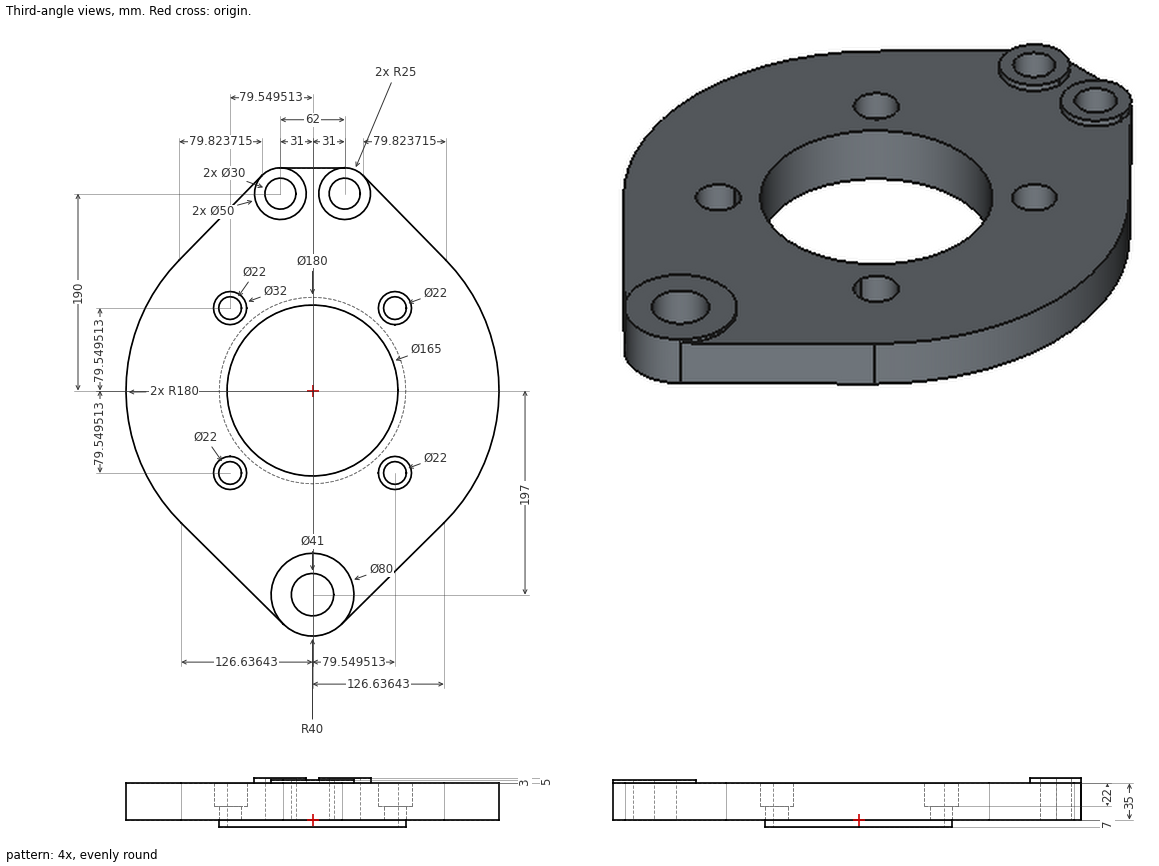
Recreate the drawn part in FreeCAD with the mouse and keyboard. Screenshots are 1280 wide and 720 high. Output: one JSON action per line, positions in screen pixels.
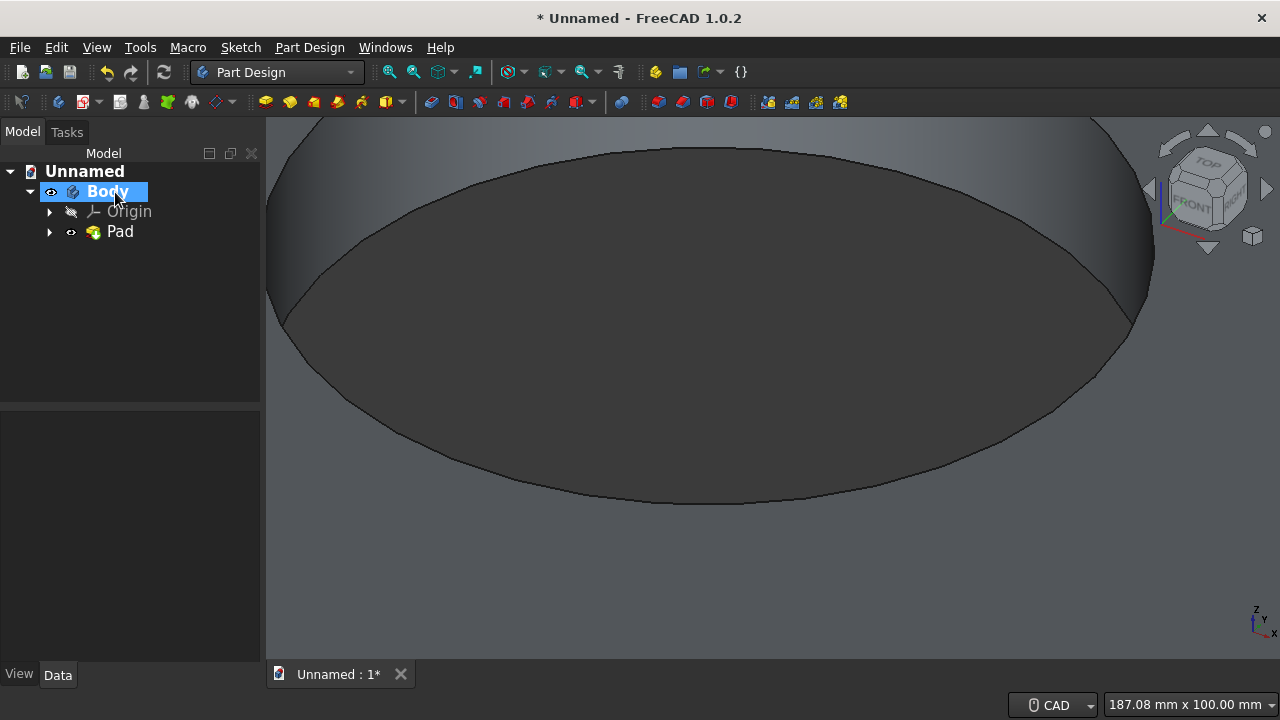
{"action": "key", "text": "v f"}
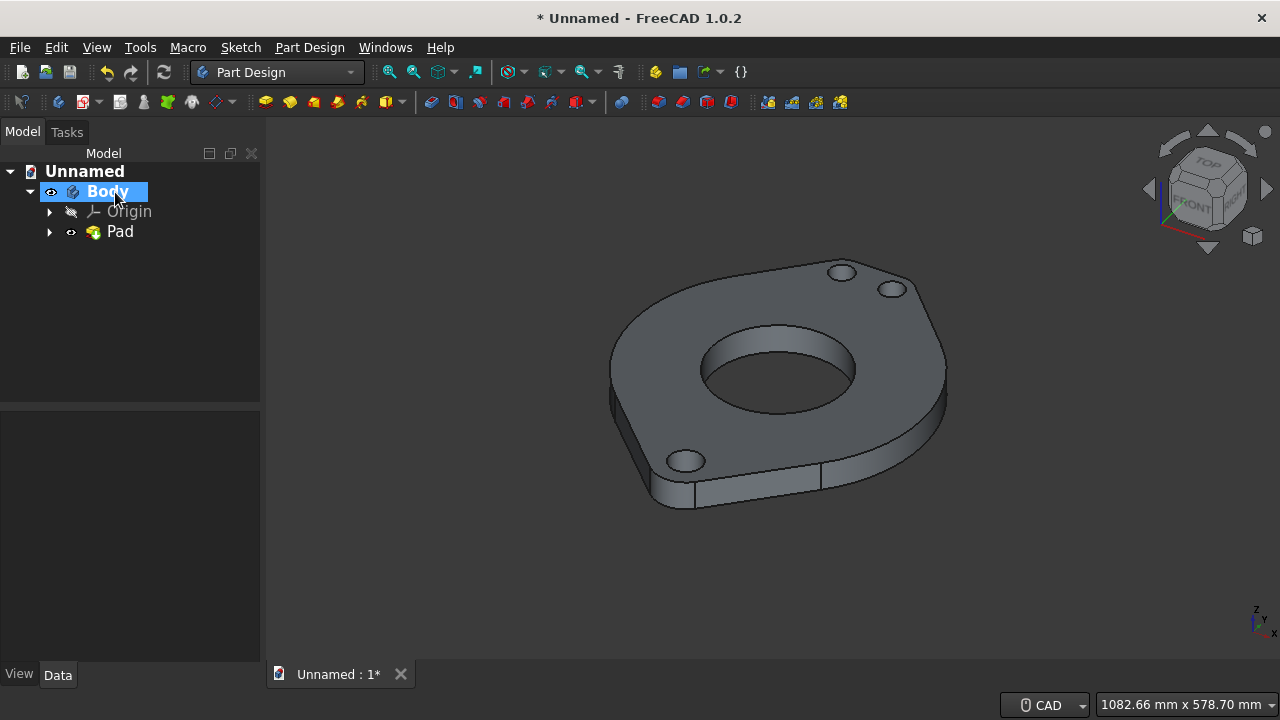
{"action": "left_click", "coordinate": [875, 327]}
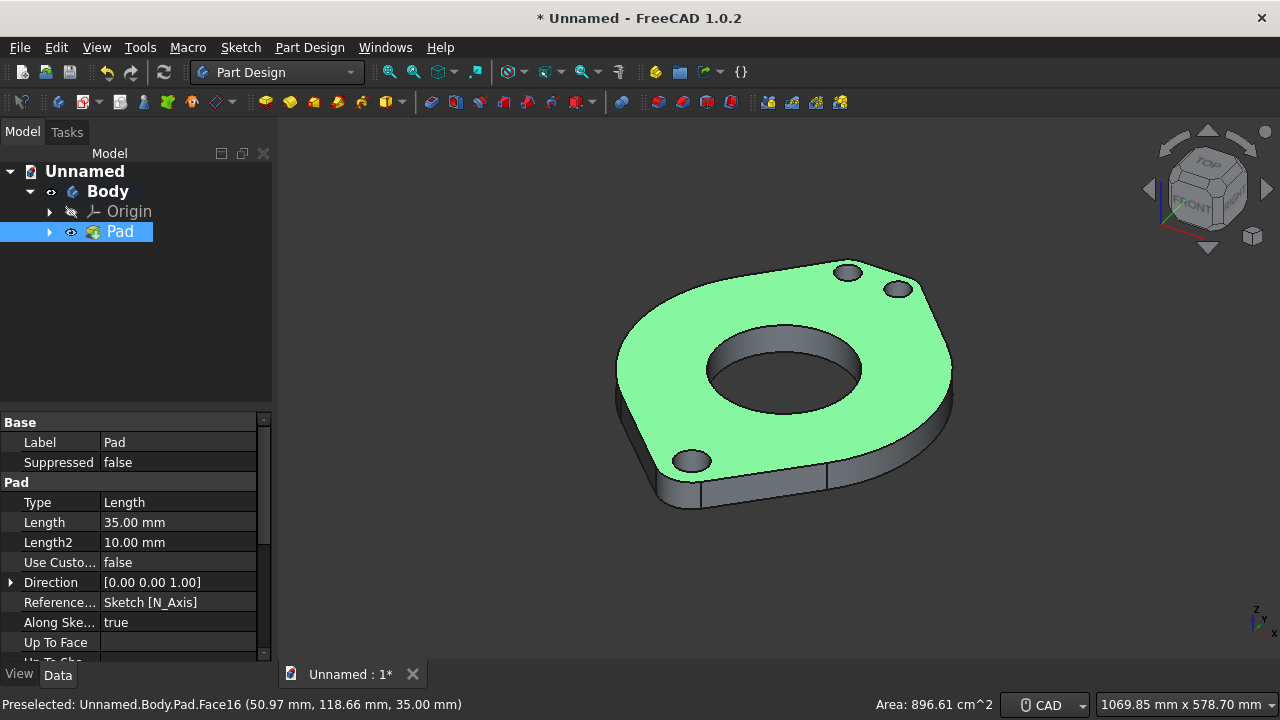
{"action": "left_click", "coordinate": [84, 102]}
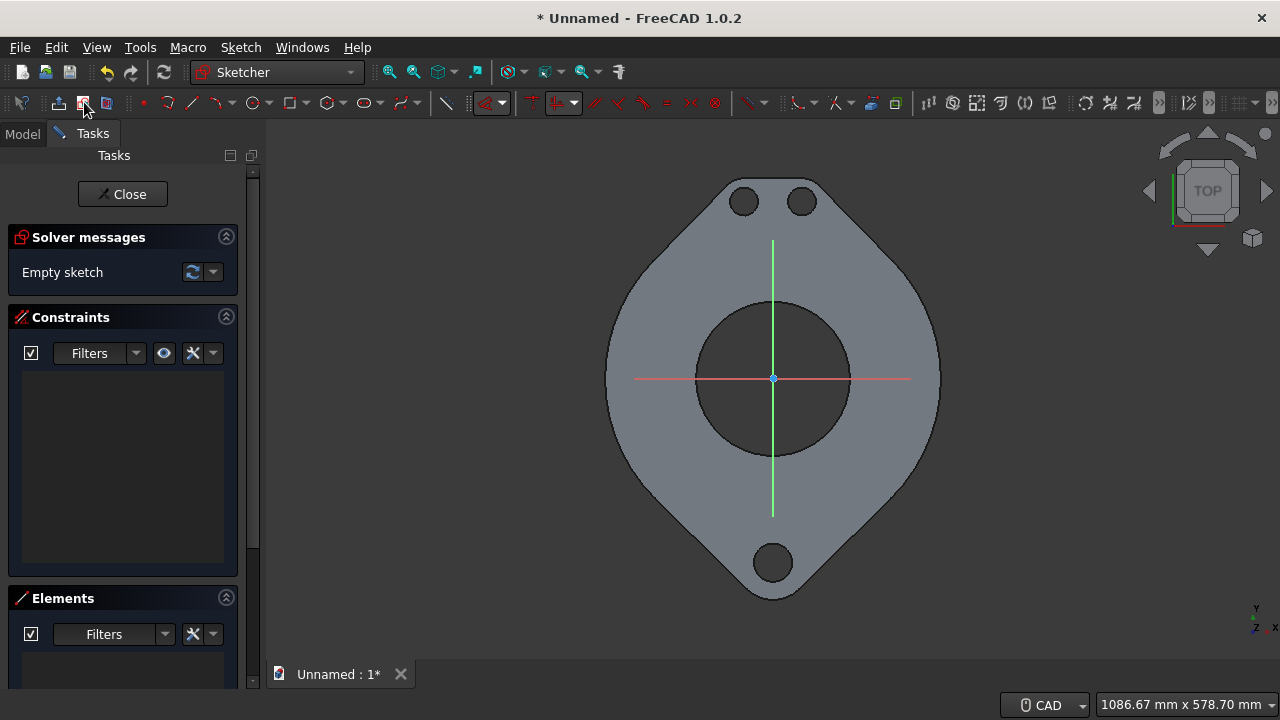
{"action": "scroll", "coordinate": [856, 147], "scroll_direction": "up", "scroll_amount": 3}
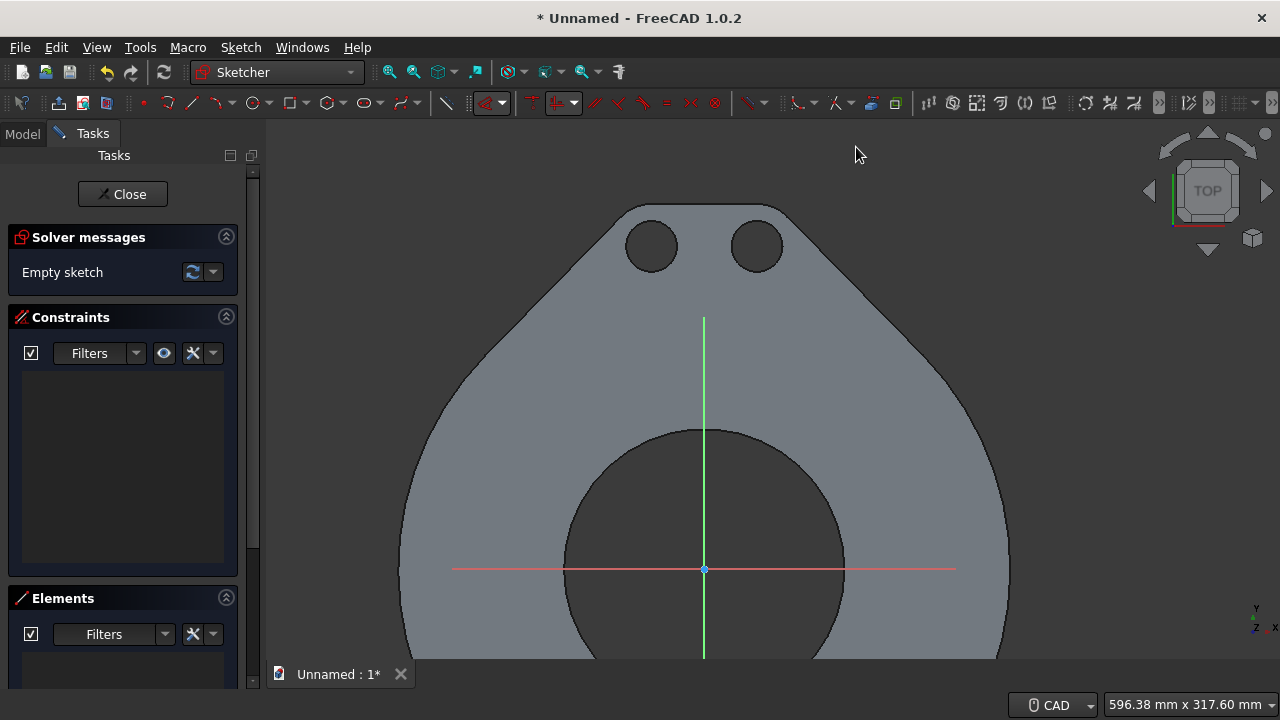
{"action": "left_click", "coordinate": [254, 104]}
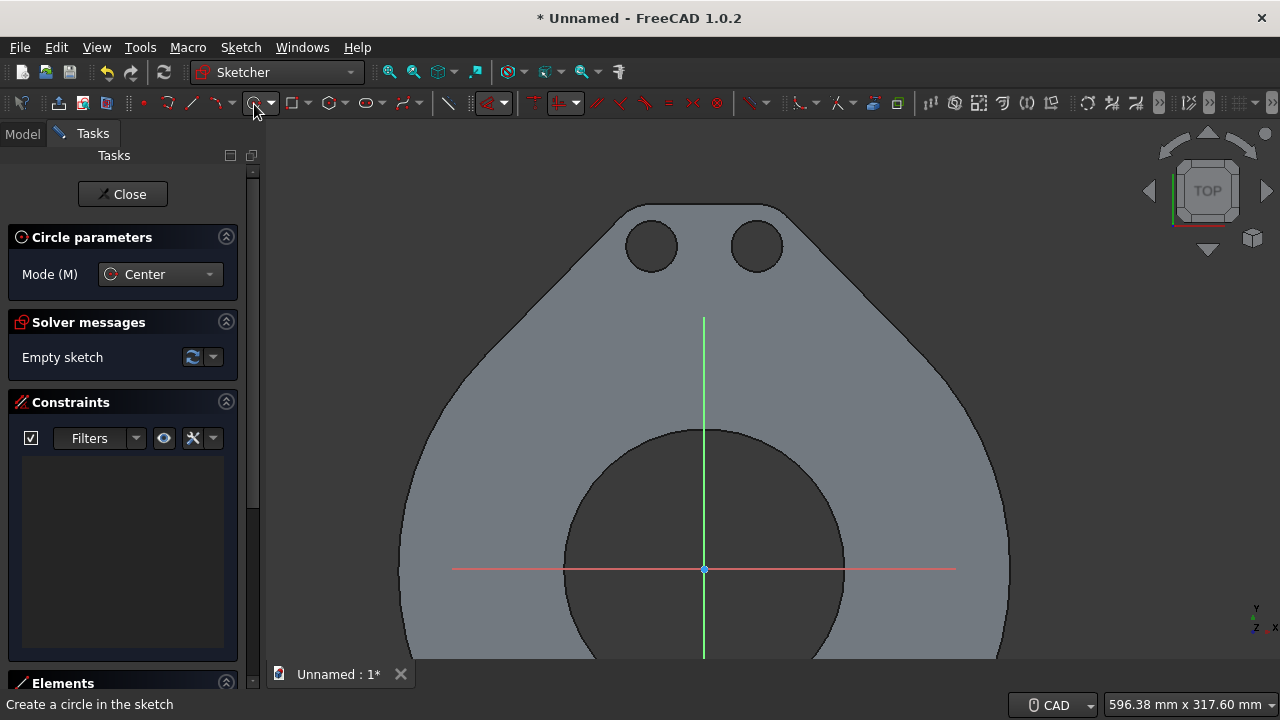
{"action": "left_click", "coordinate": [652, 246]}
{"action": "left_click", "coordinate": [682, 216]}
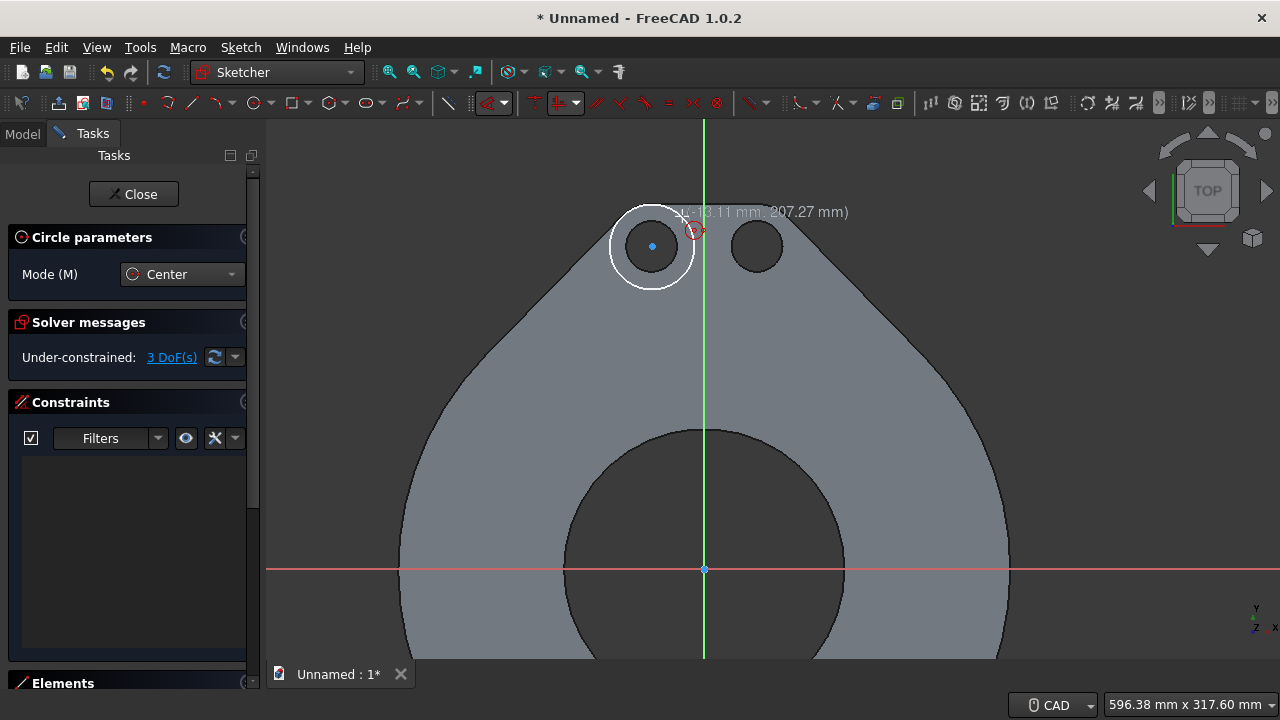
{"action": "left_click", "coordinate": [757, 246]}
{"action": "left_click", "coordinate": [787, 216]}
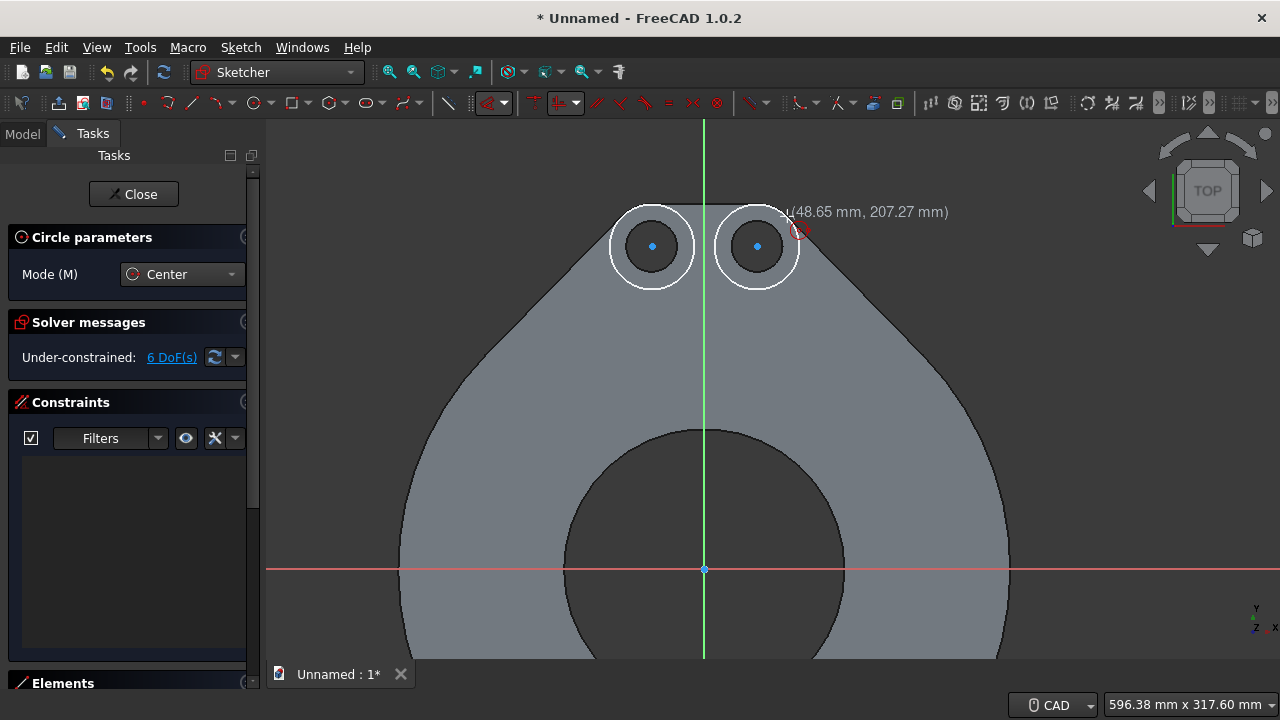
{"action": "left_click", "coordinate": [652, 247]}
{"action": "left_click", "coordinate": [670, 228]}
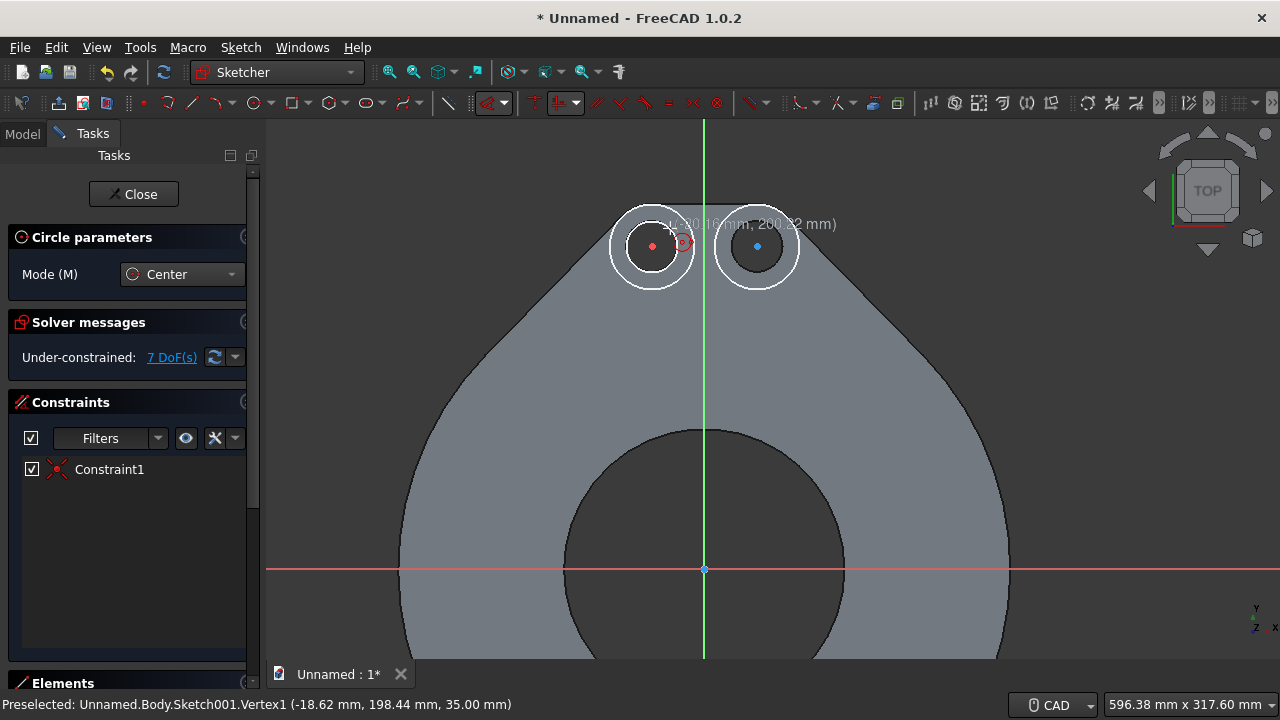
{"action": "left_click", "coordinate": [757, 247]}
{"action": "left_click", "coordinate": [775, 228]}
{"action": "key", "text": "Escape"}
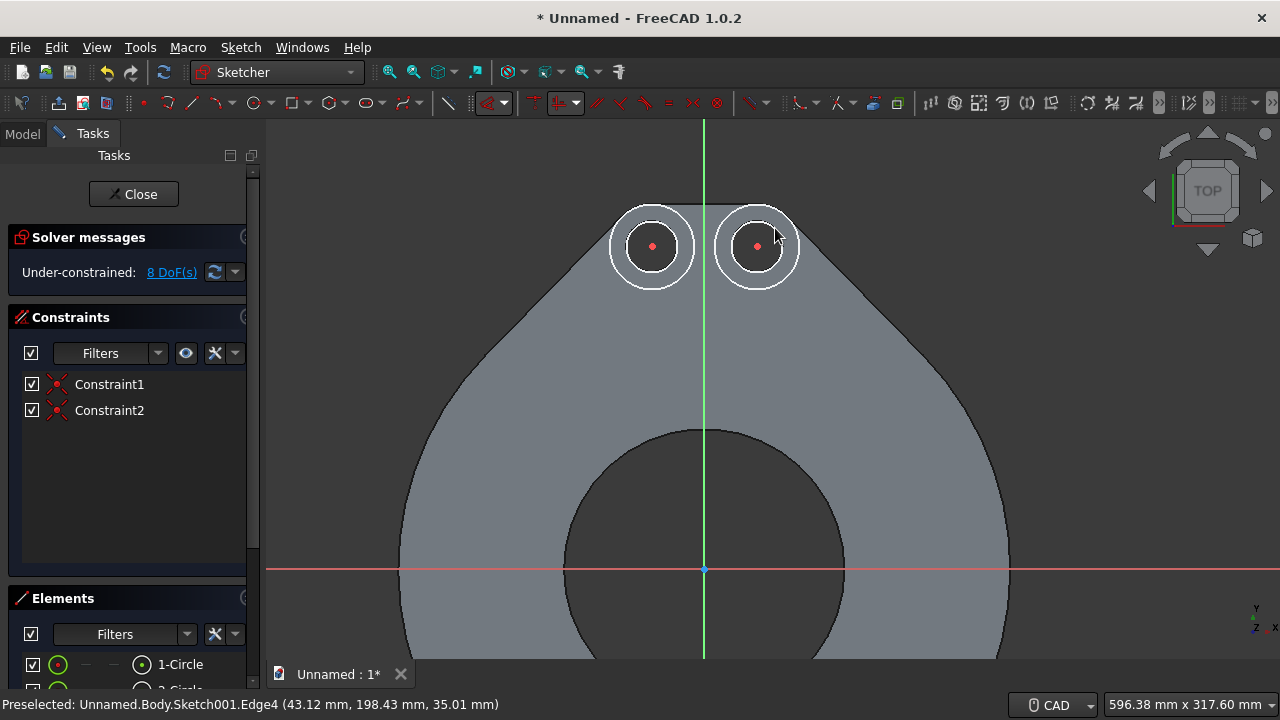
{"action": "left_click", "coordinate": [682, 217]}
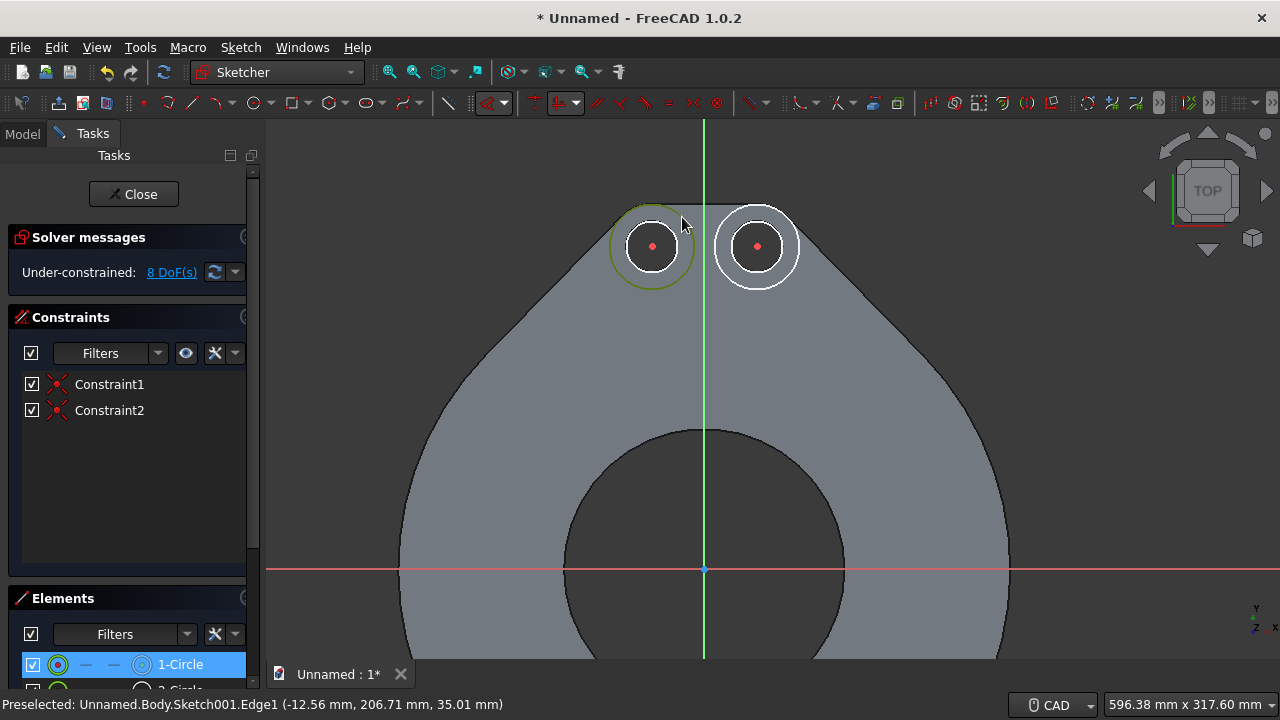
{"action": "left_click", "coordinate": [787, 217]}